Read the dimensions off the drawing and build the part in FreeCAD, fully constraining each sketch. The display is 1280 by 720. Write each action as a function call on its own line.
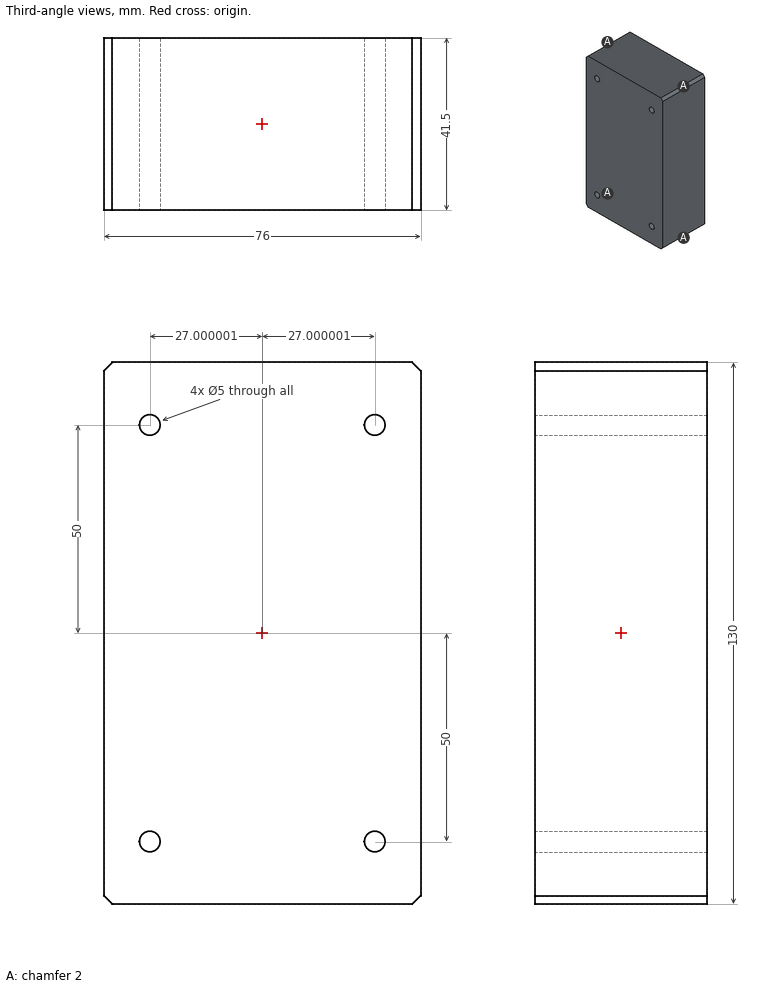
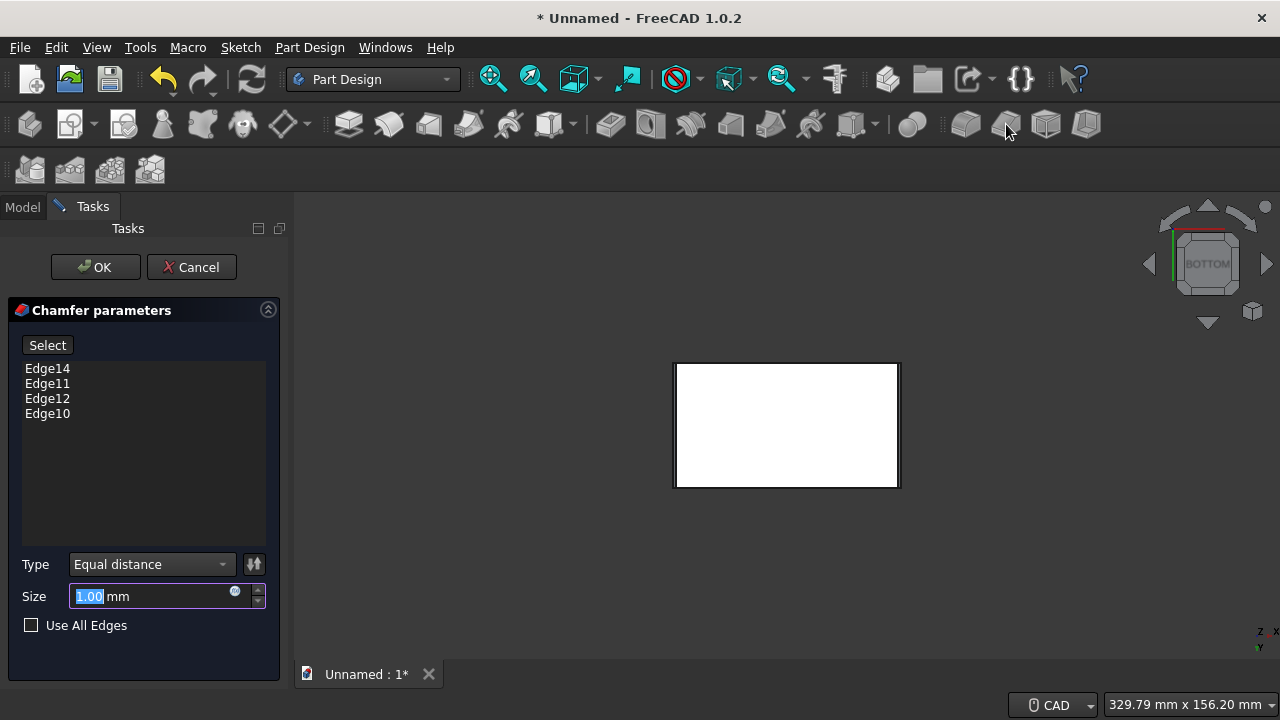
text(2)
key(Tab)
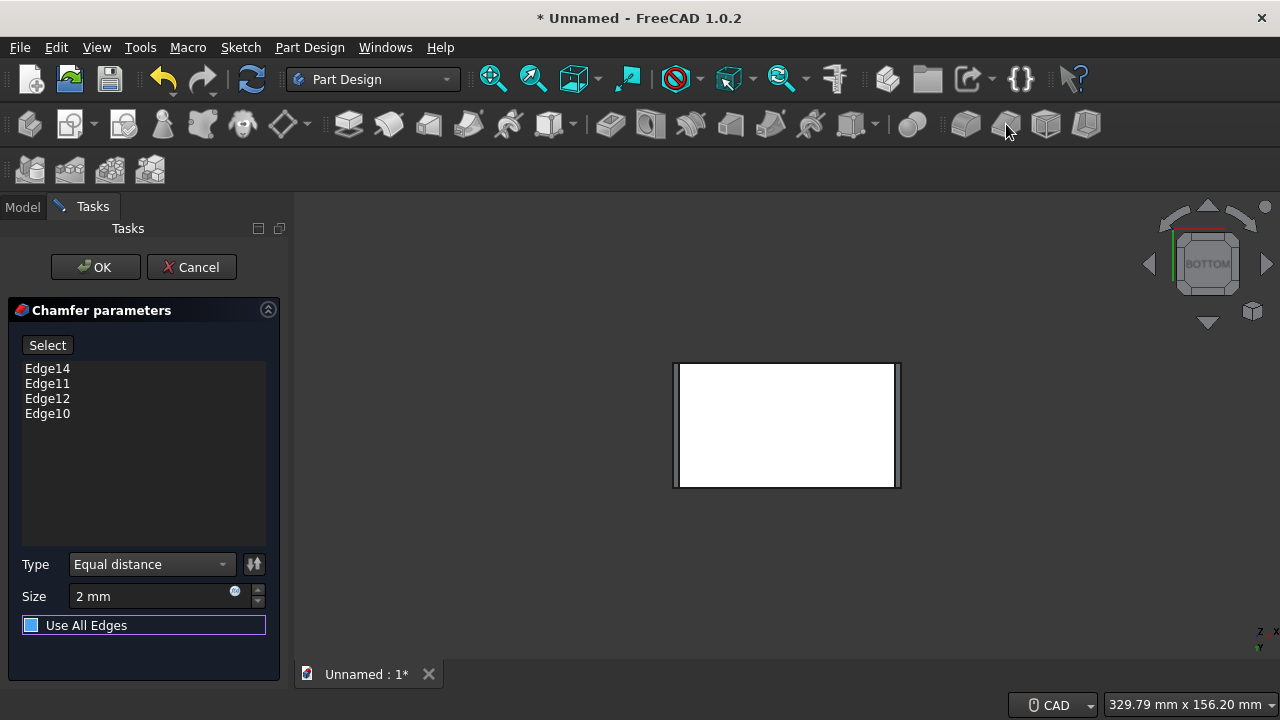
click(96, 267)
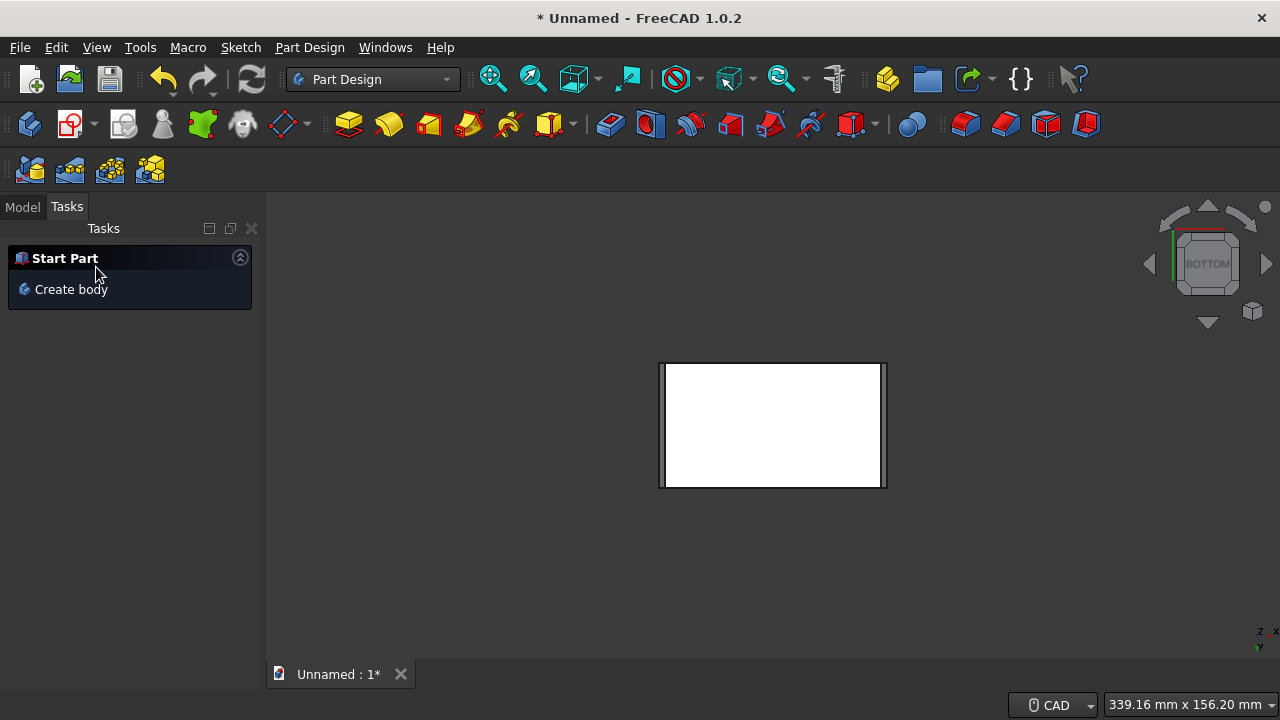
key(0)